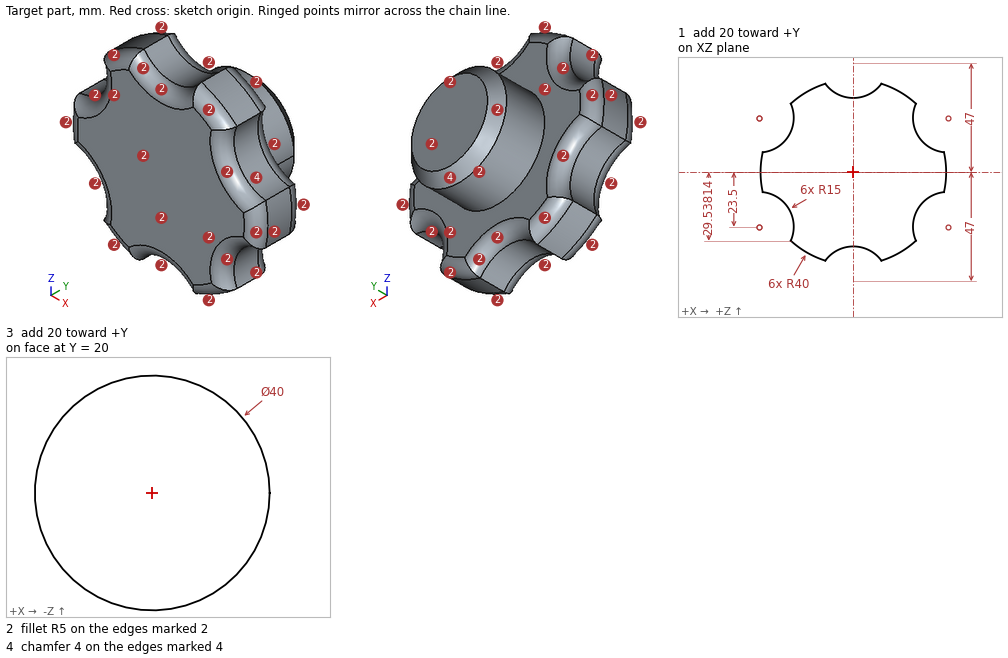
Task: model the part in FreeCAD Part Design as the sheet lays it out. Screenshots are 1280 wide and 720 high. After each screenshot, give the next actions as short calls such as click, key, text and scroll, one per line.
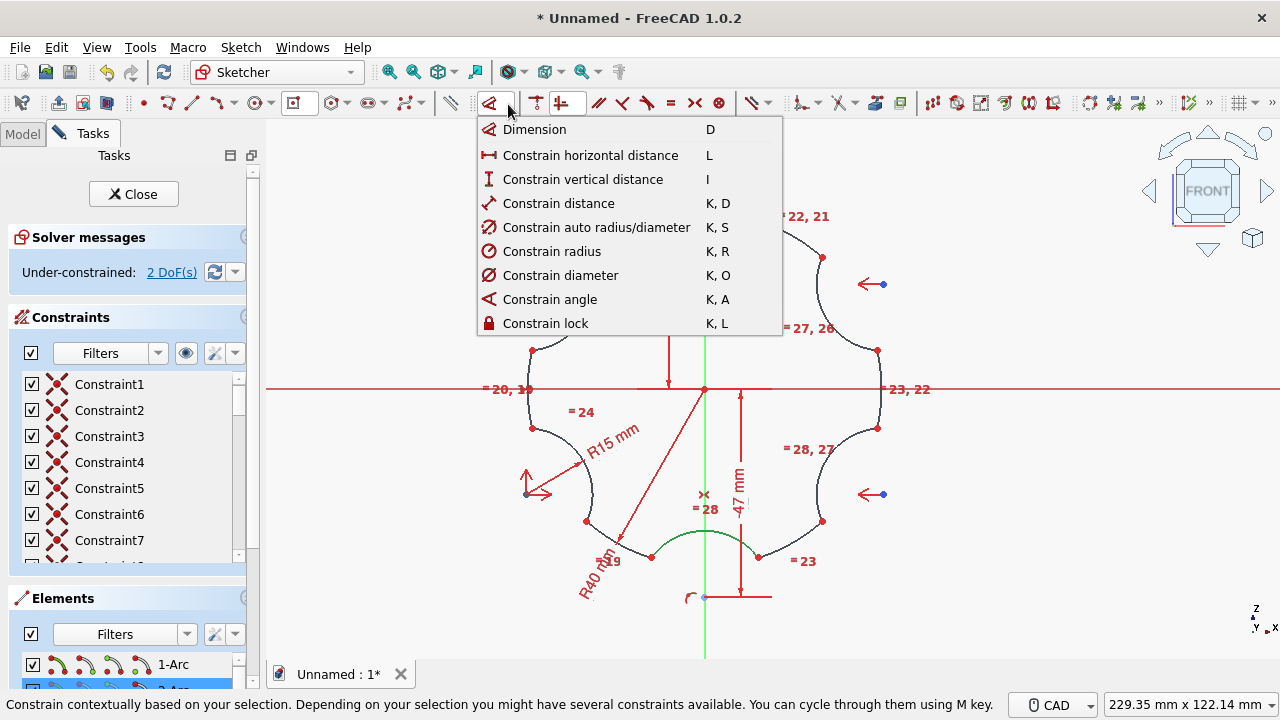
click(630, 179)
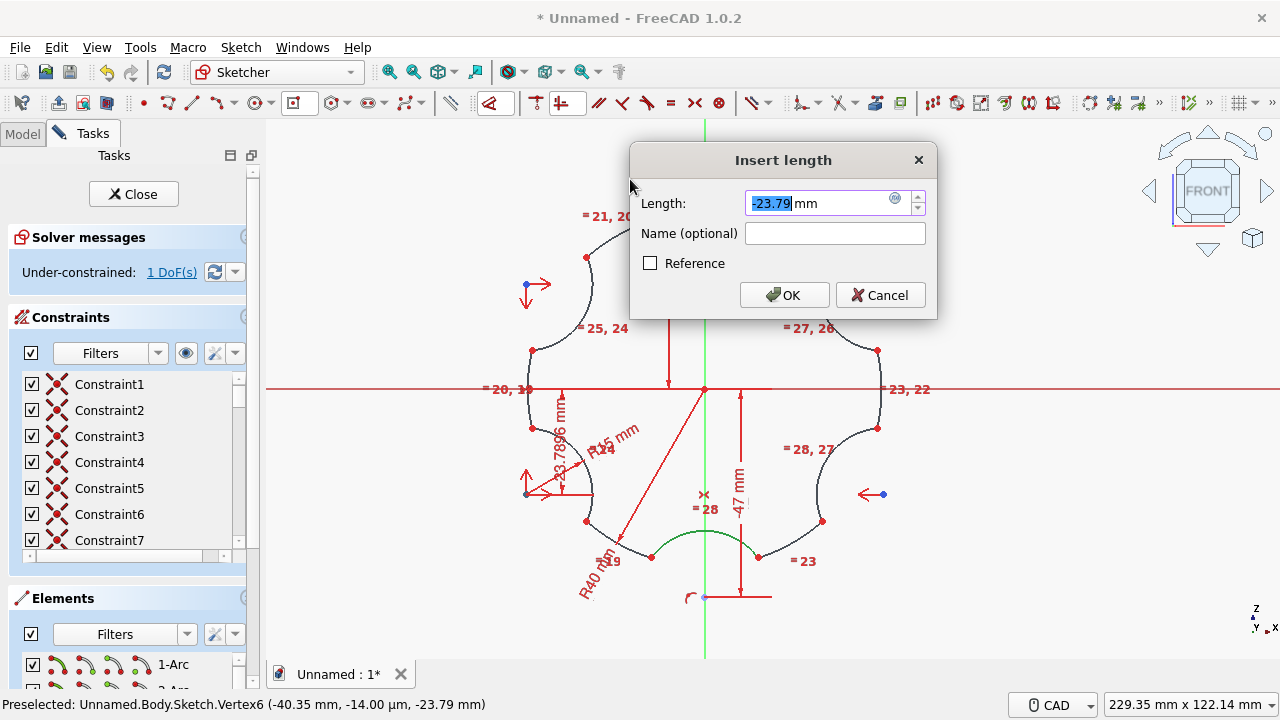
text(-23.5)
key(Return)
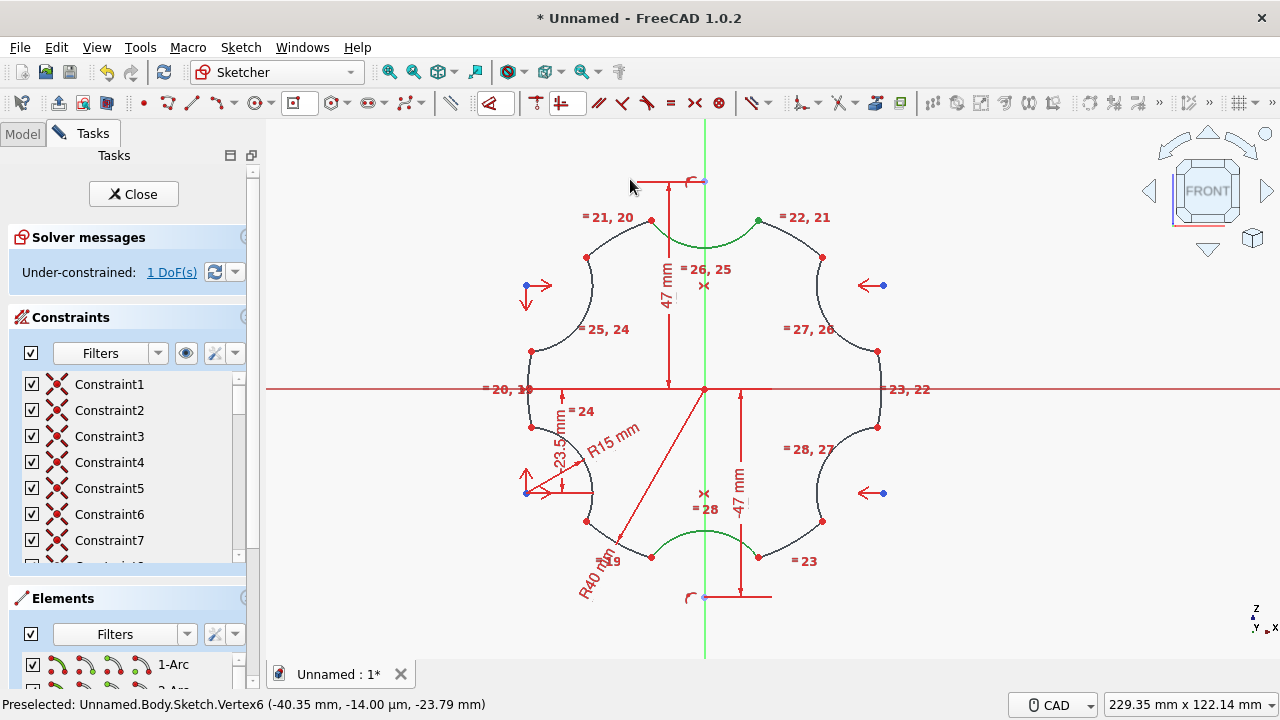
click(586, 521)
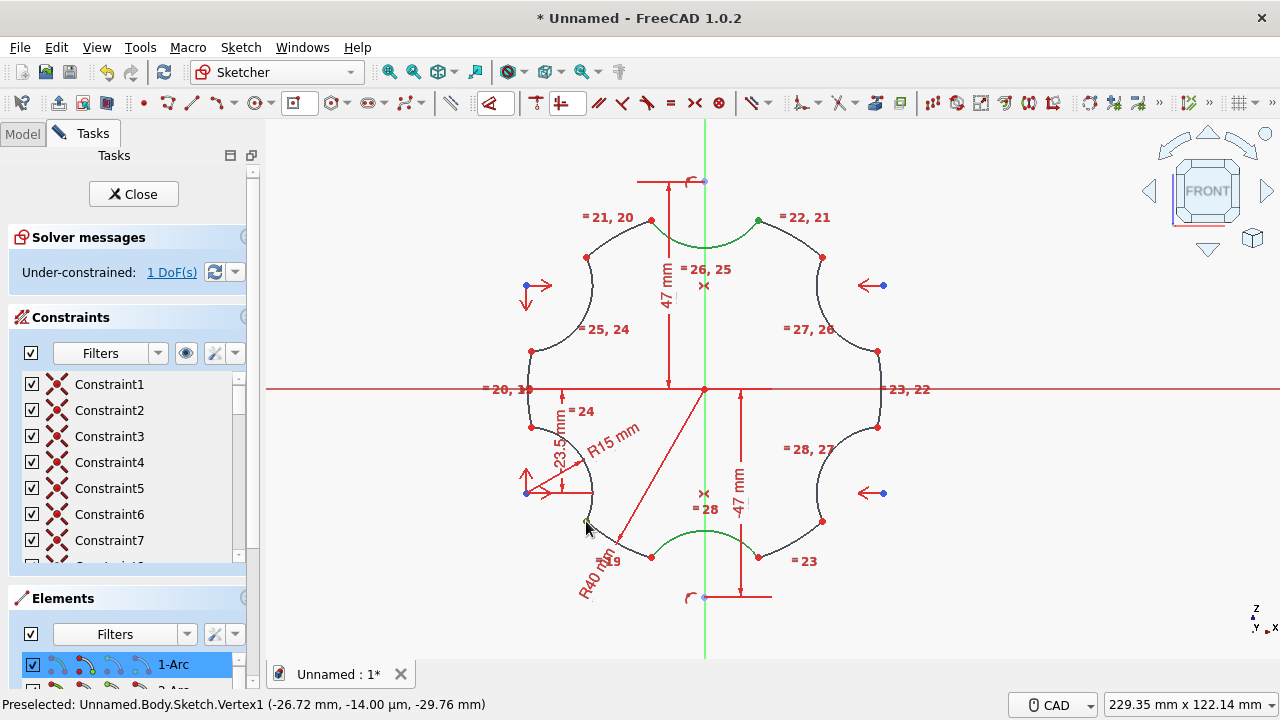
key(i)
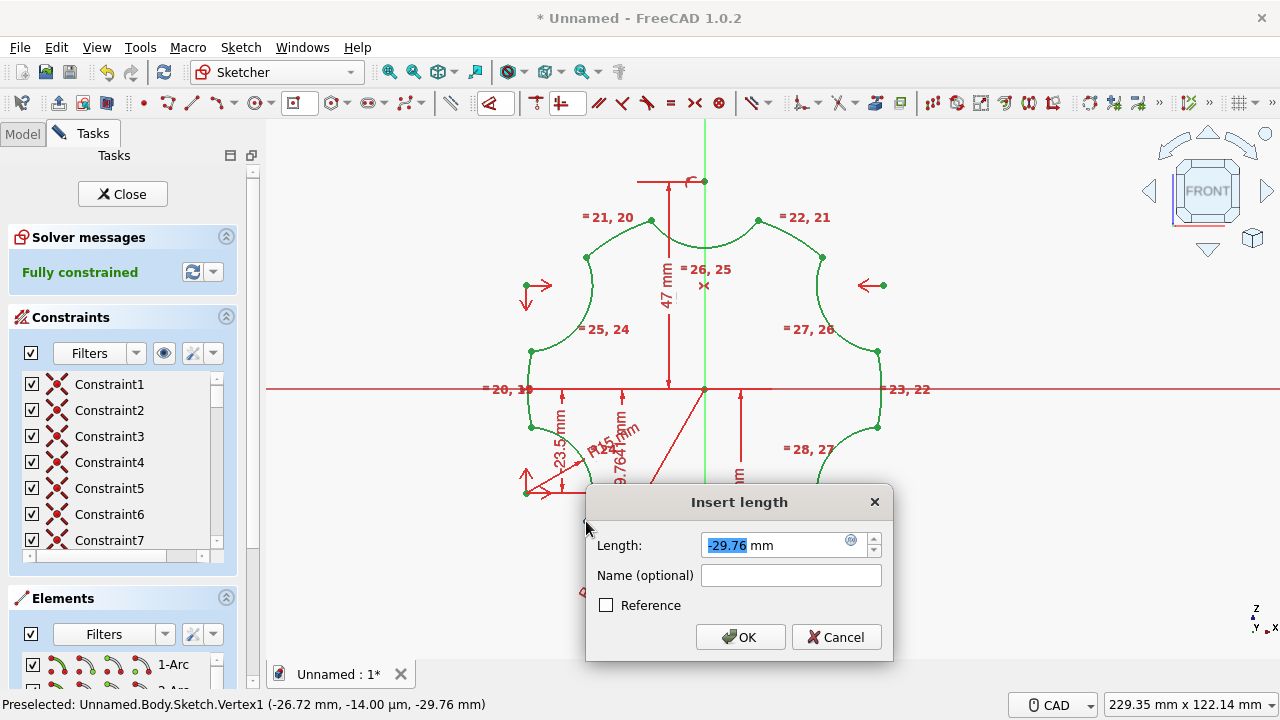
text(-29.53814)
key(Return)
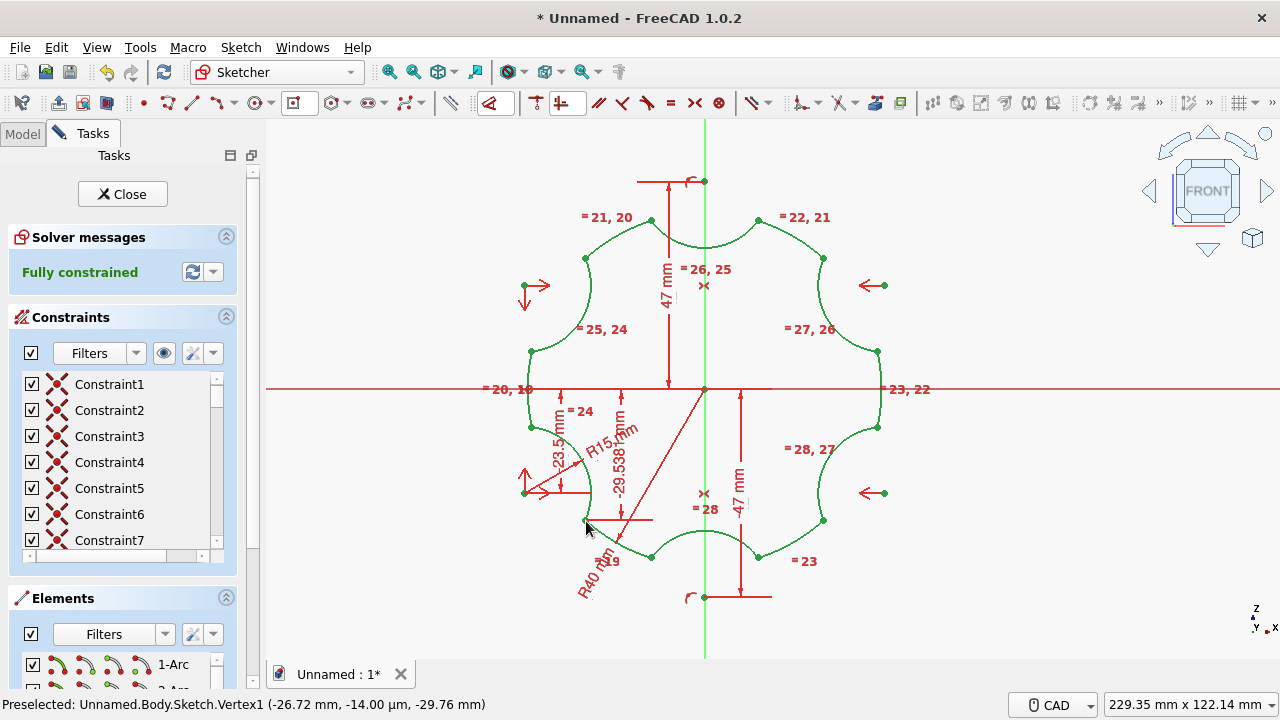
click(123, 194)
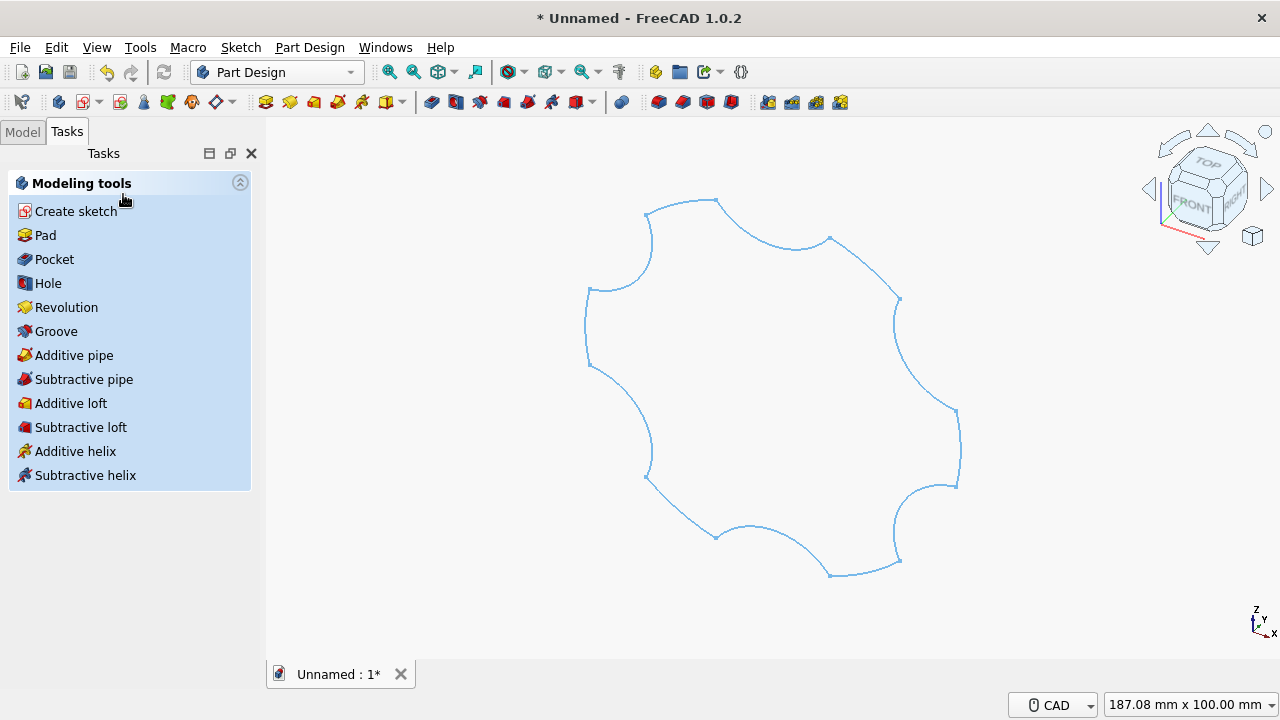
click(266, 102)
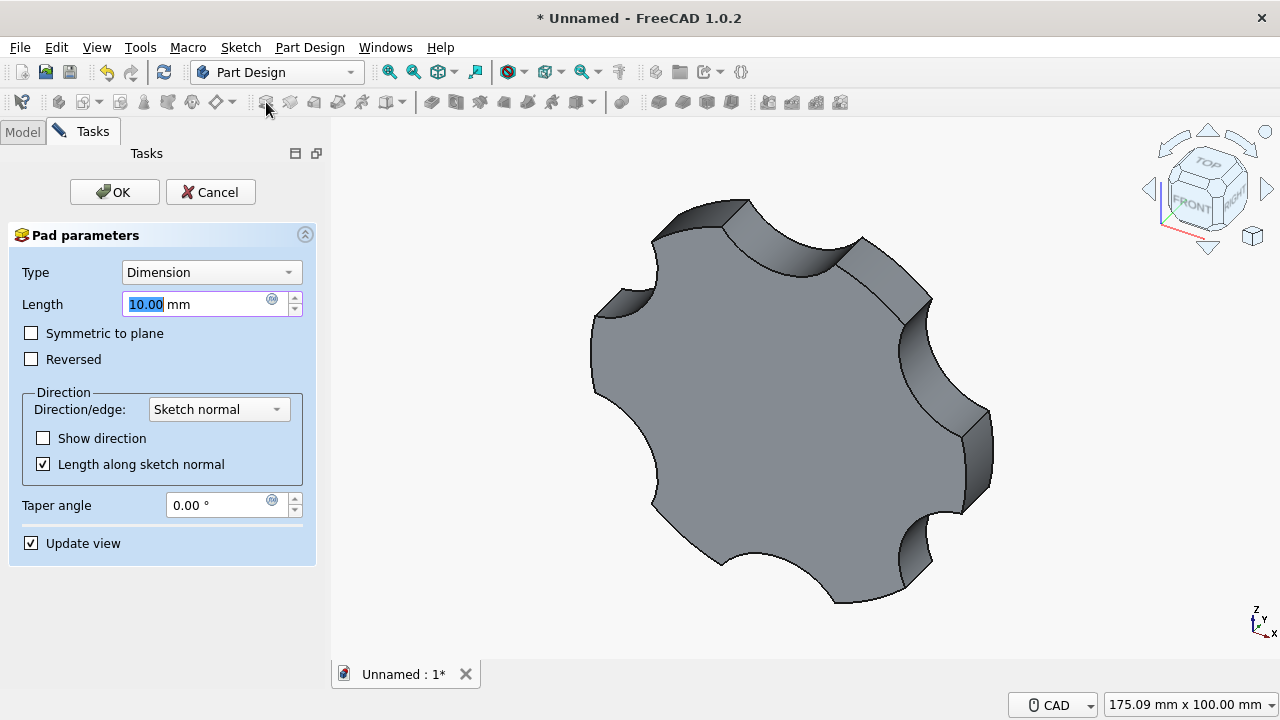
text(20)
key(Tab)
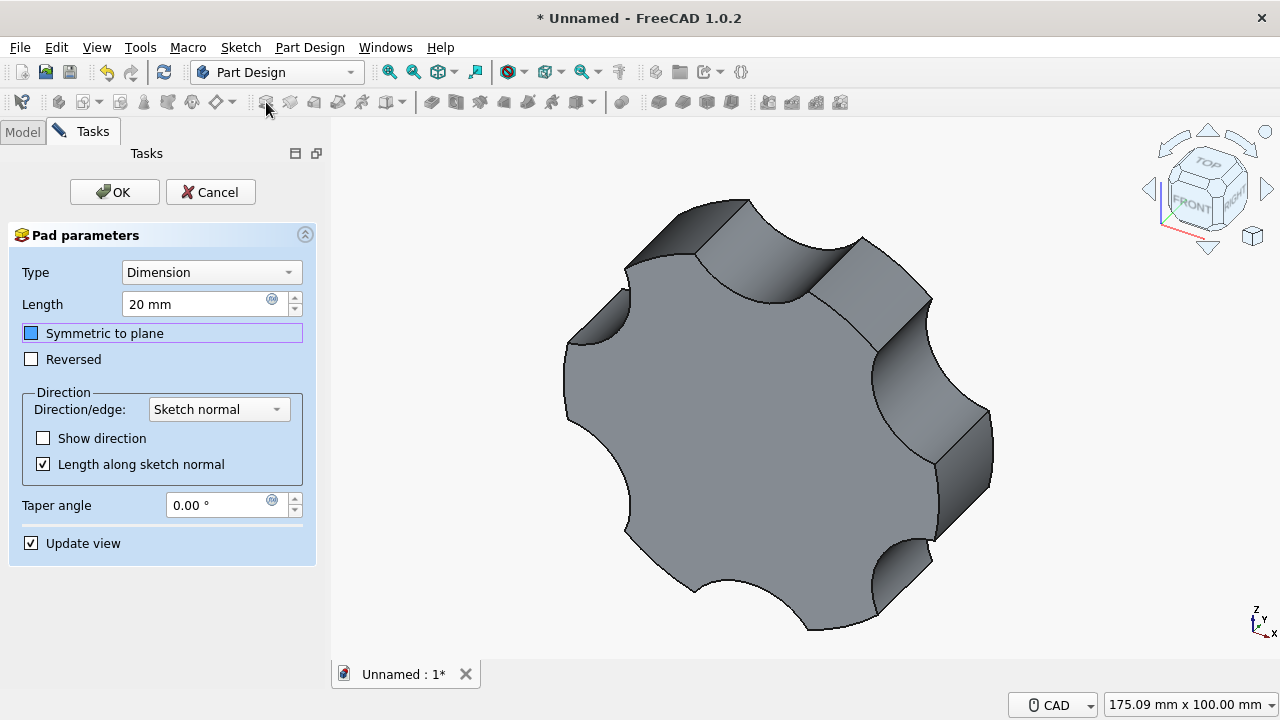
click(30, 359)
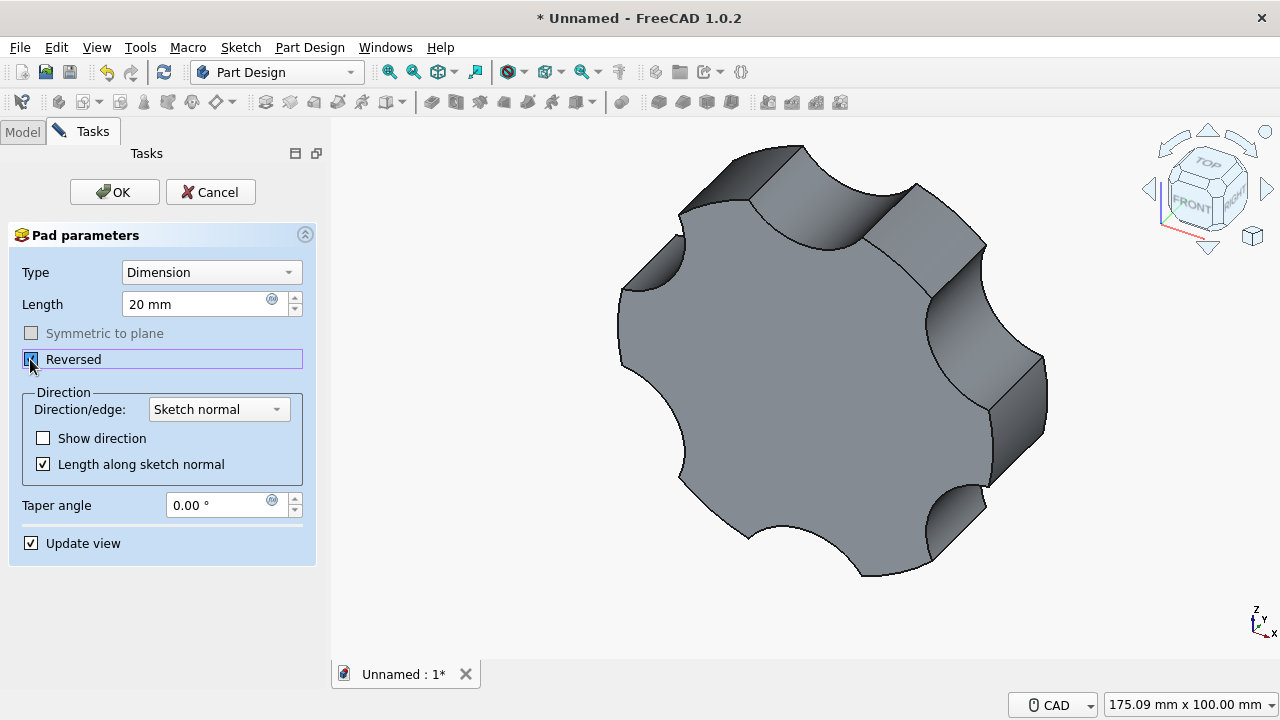
click(115, 192)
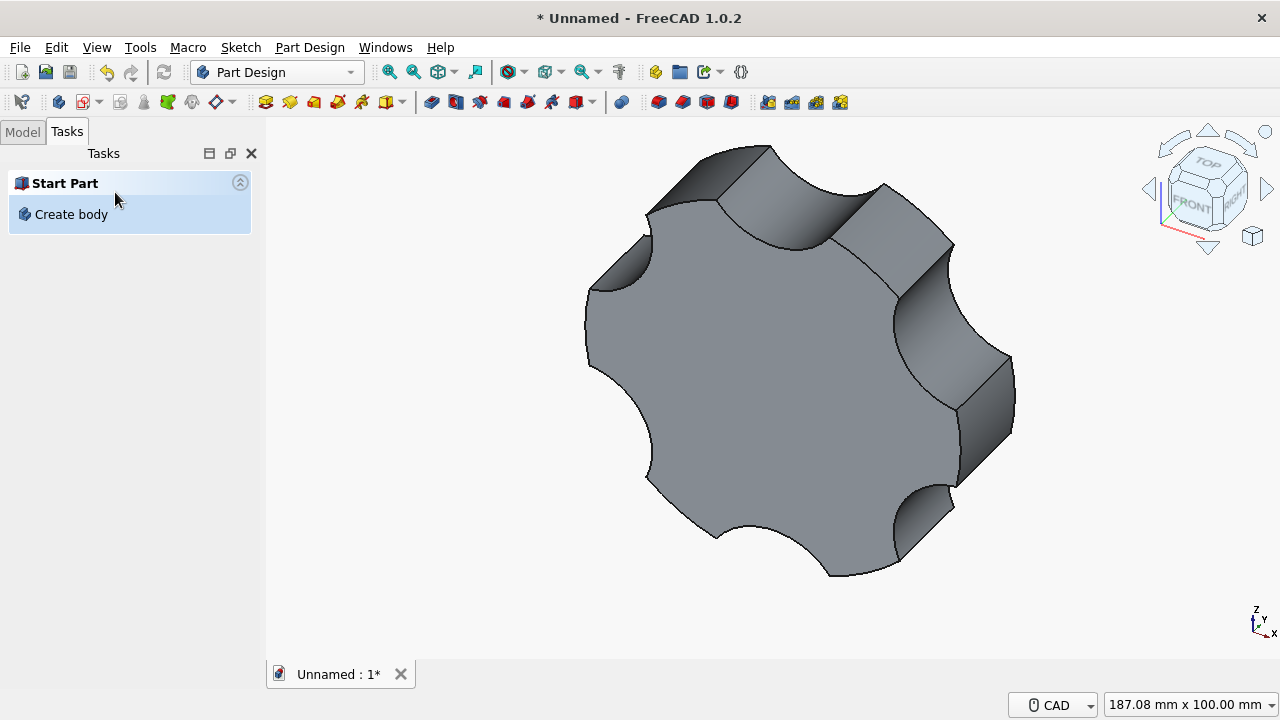
click(390, 72)